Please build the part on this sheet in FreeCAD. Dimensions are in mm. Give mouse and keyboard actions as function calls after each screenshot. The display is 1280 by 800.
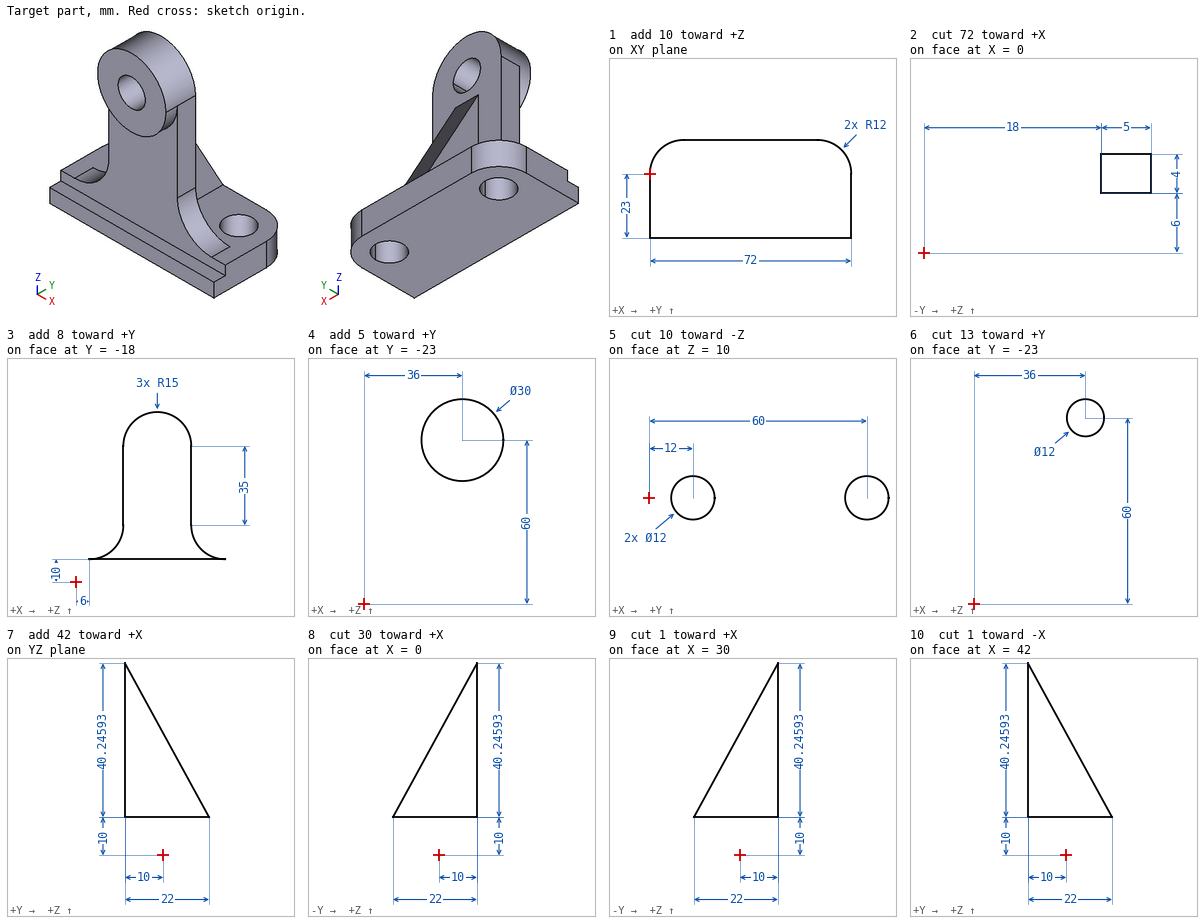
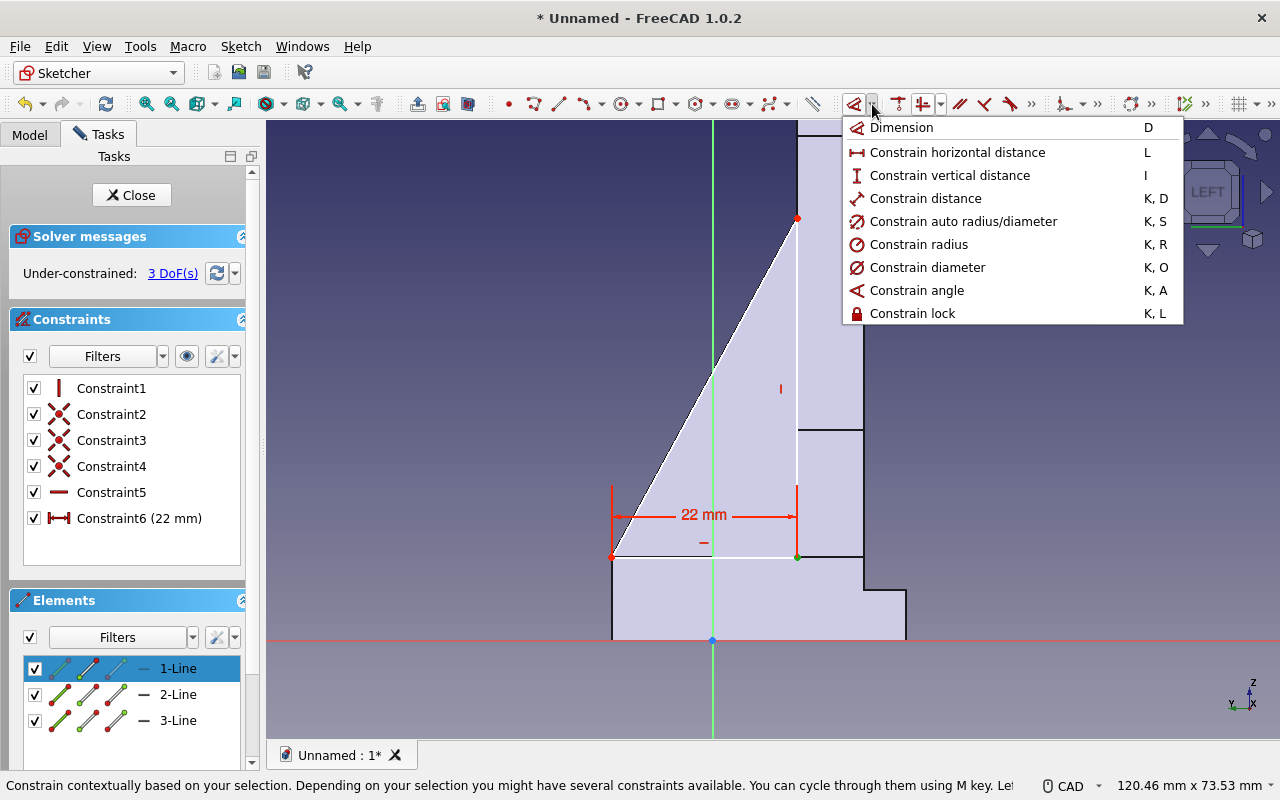
click(1013, 152)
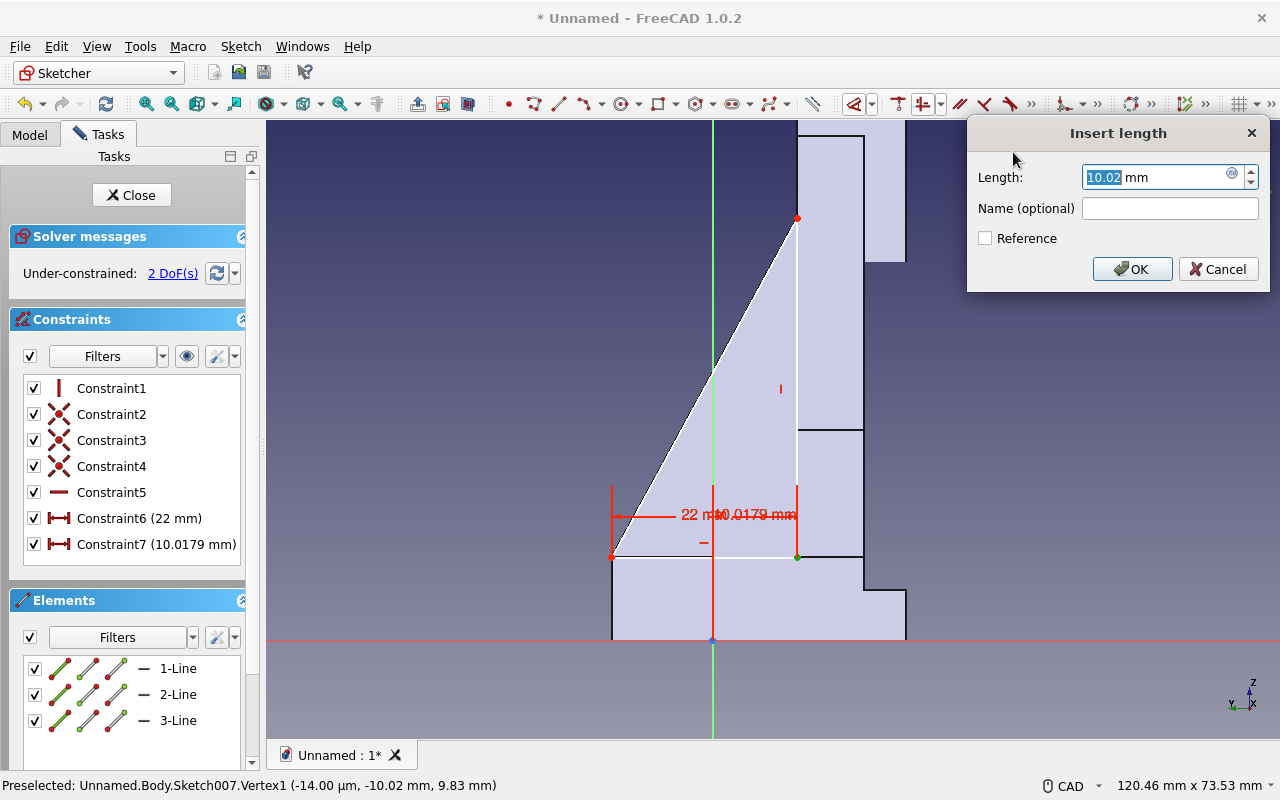
text(10)
key(Return)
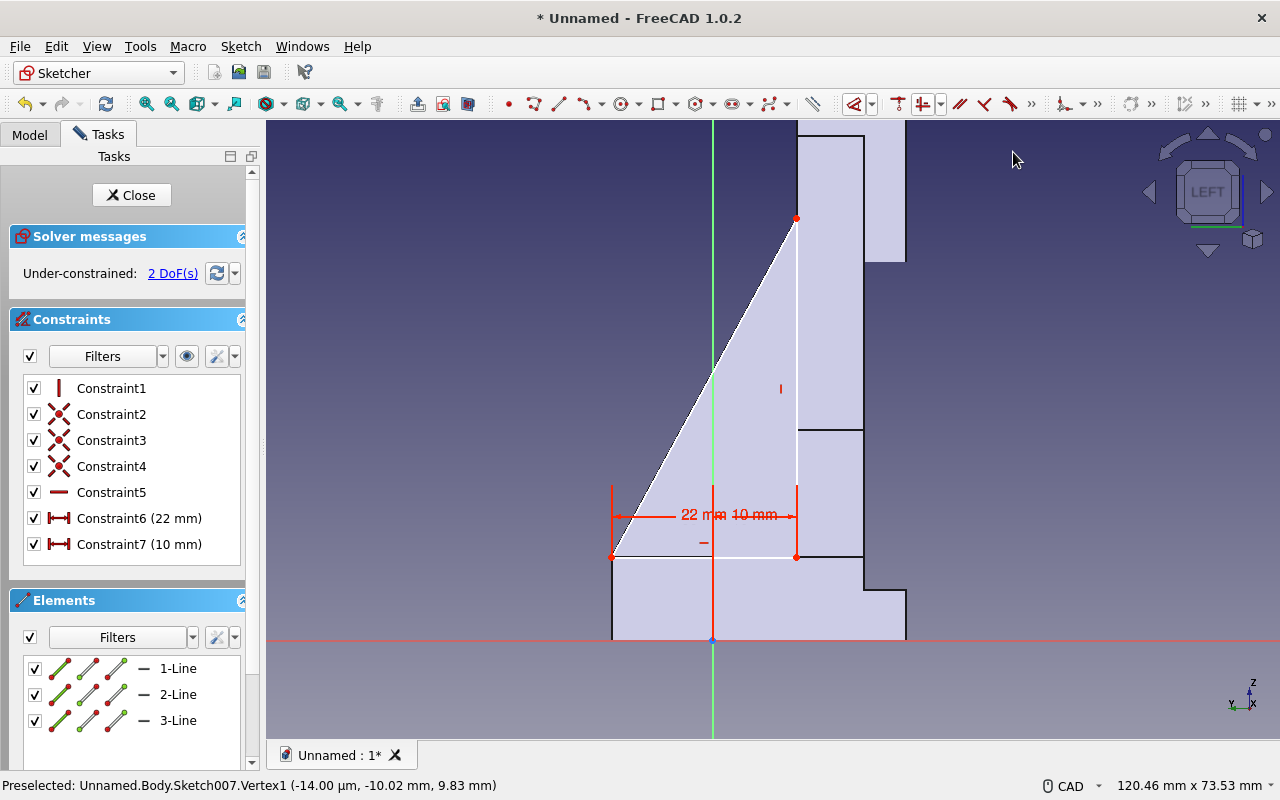
click(797, 558)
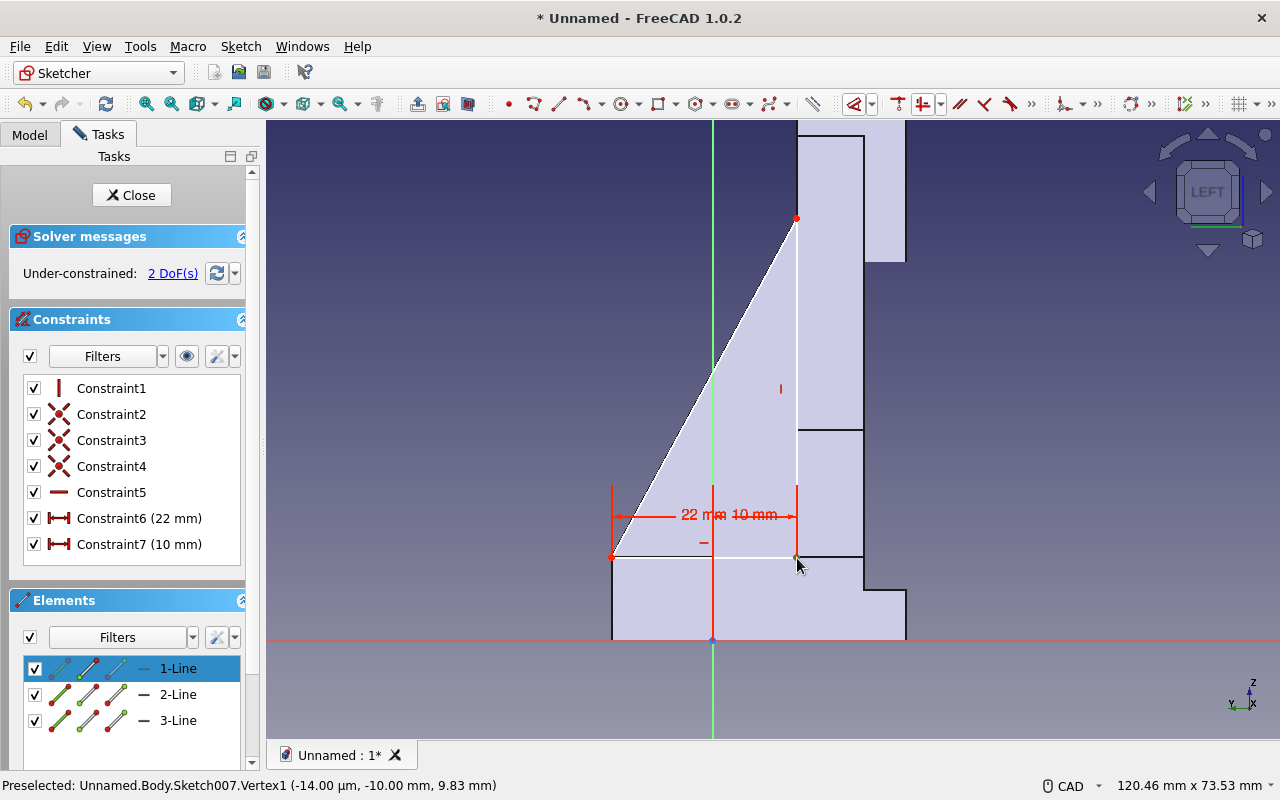
key(i)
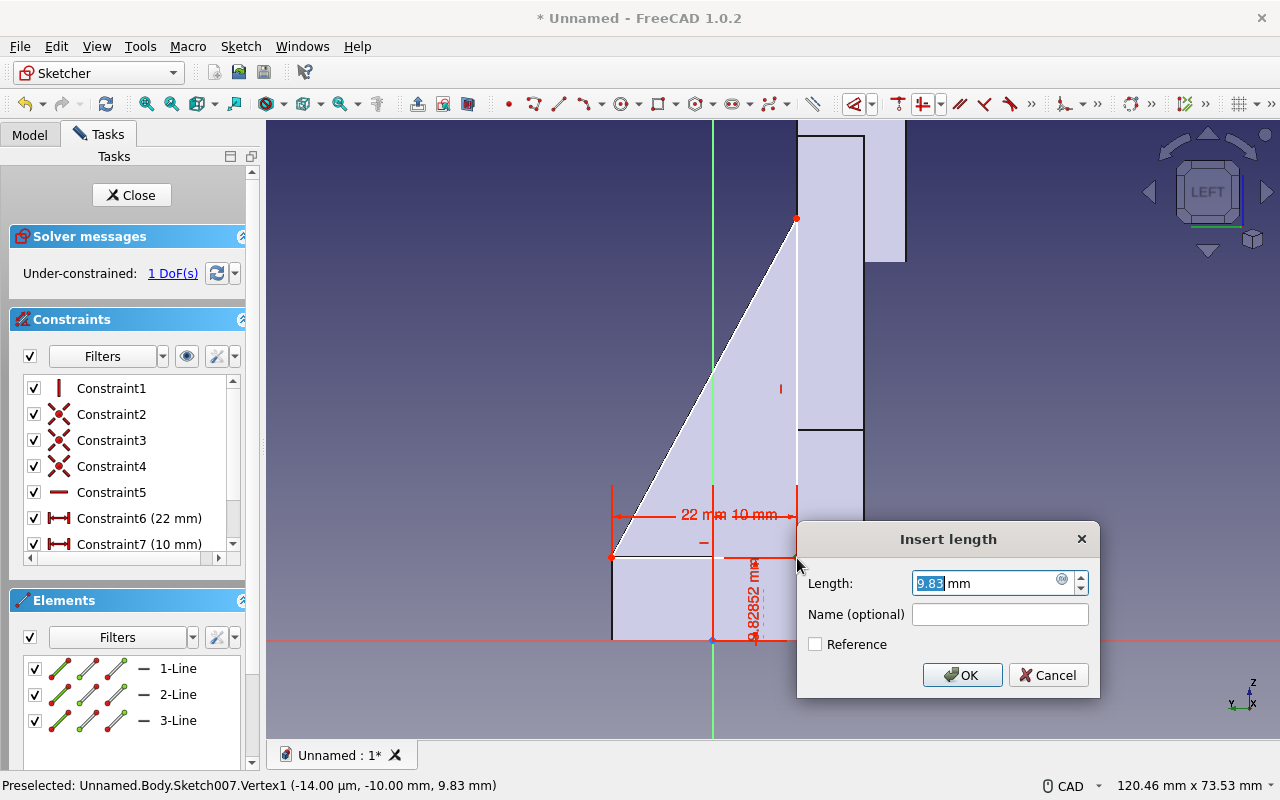
text(10)
key(Return)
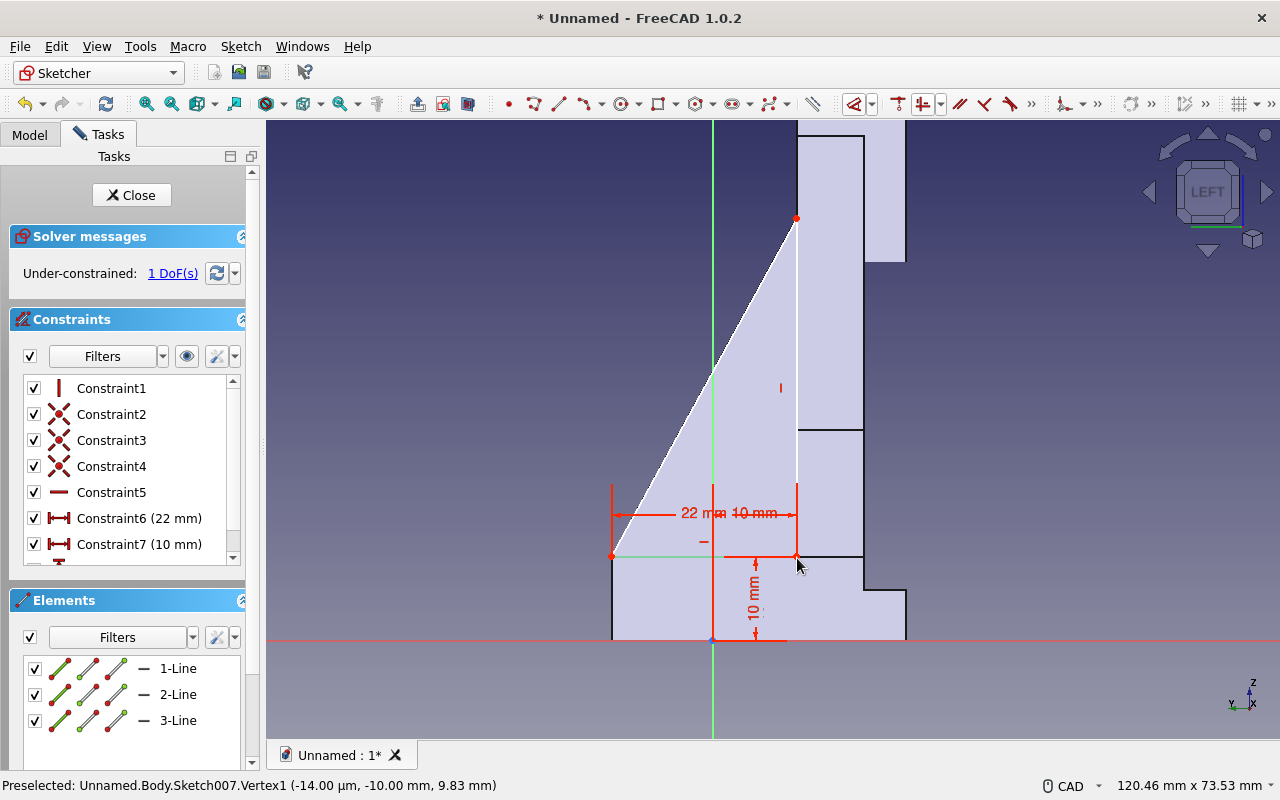
click(797, 455)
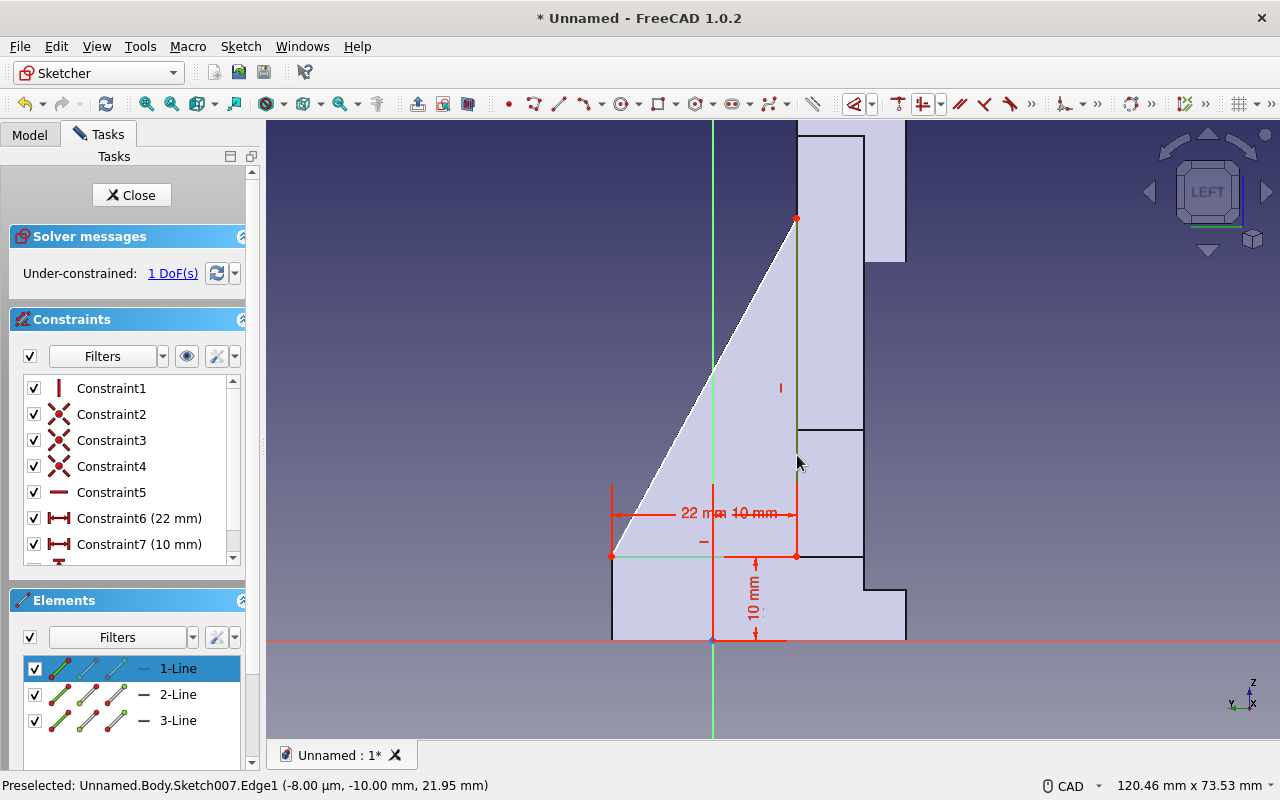
click(872, 104)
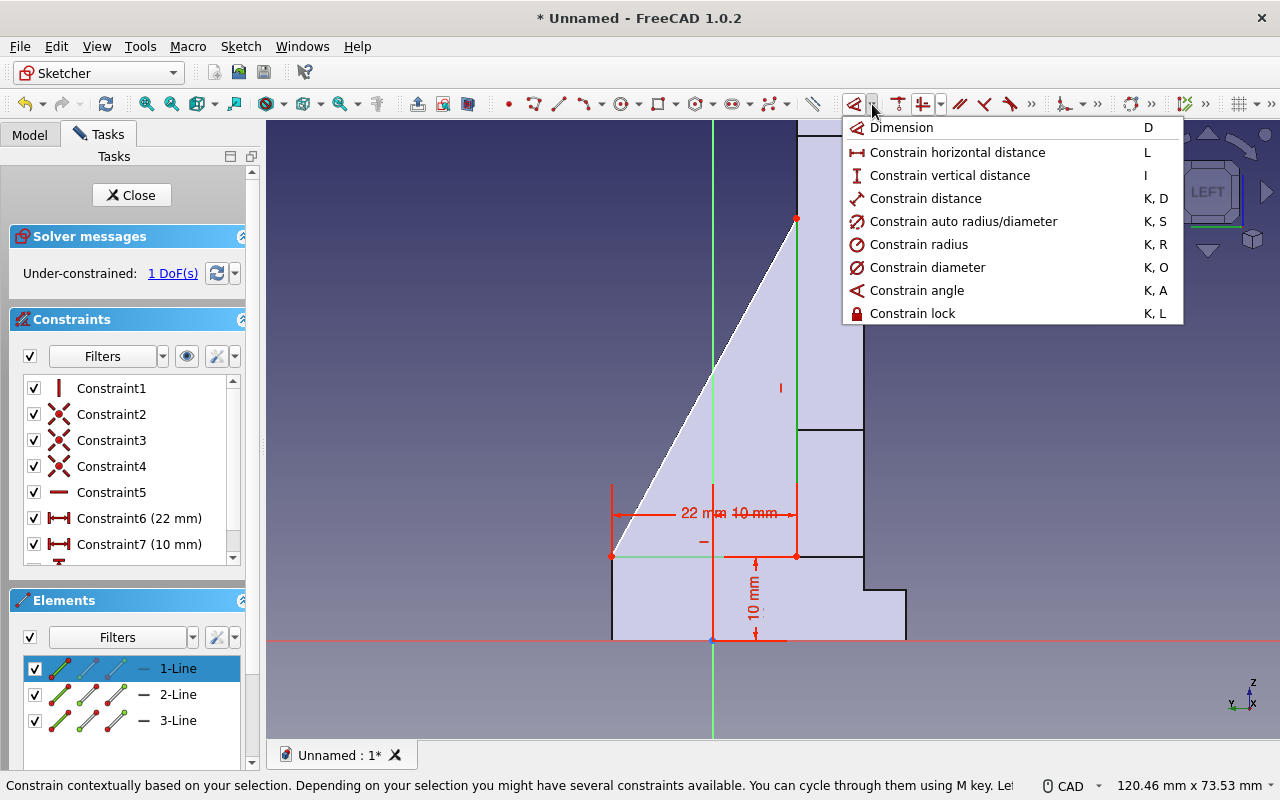
click(1013, 176)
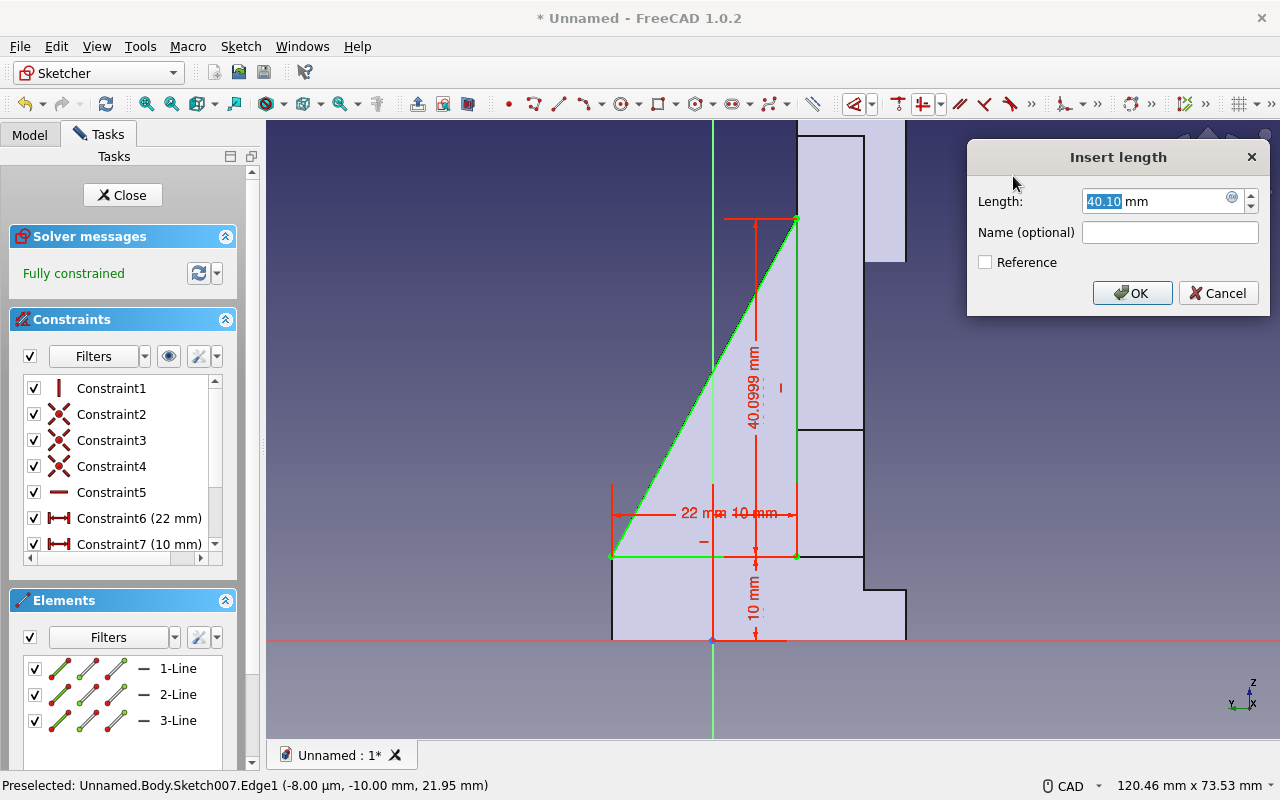
text(40.24593)
key(Return)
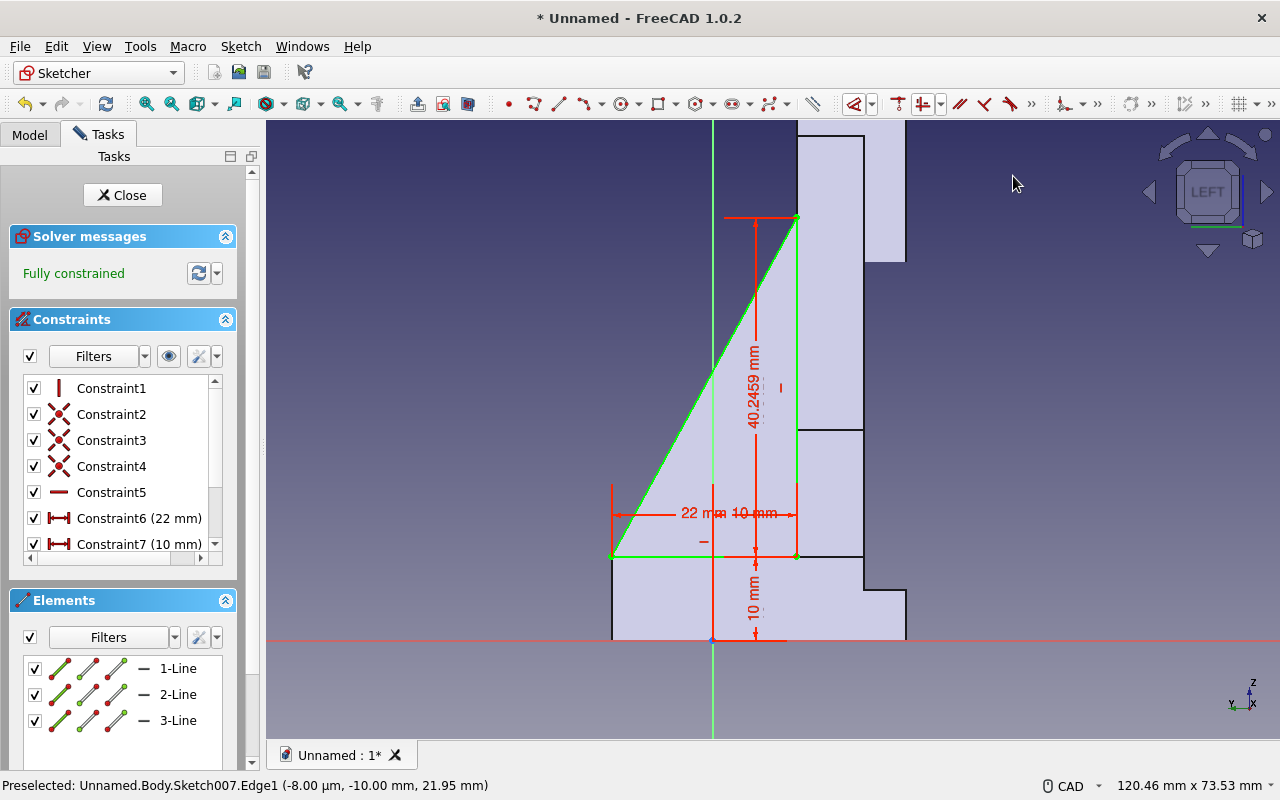
click(123, 195)